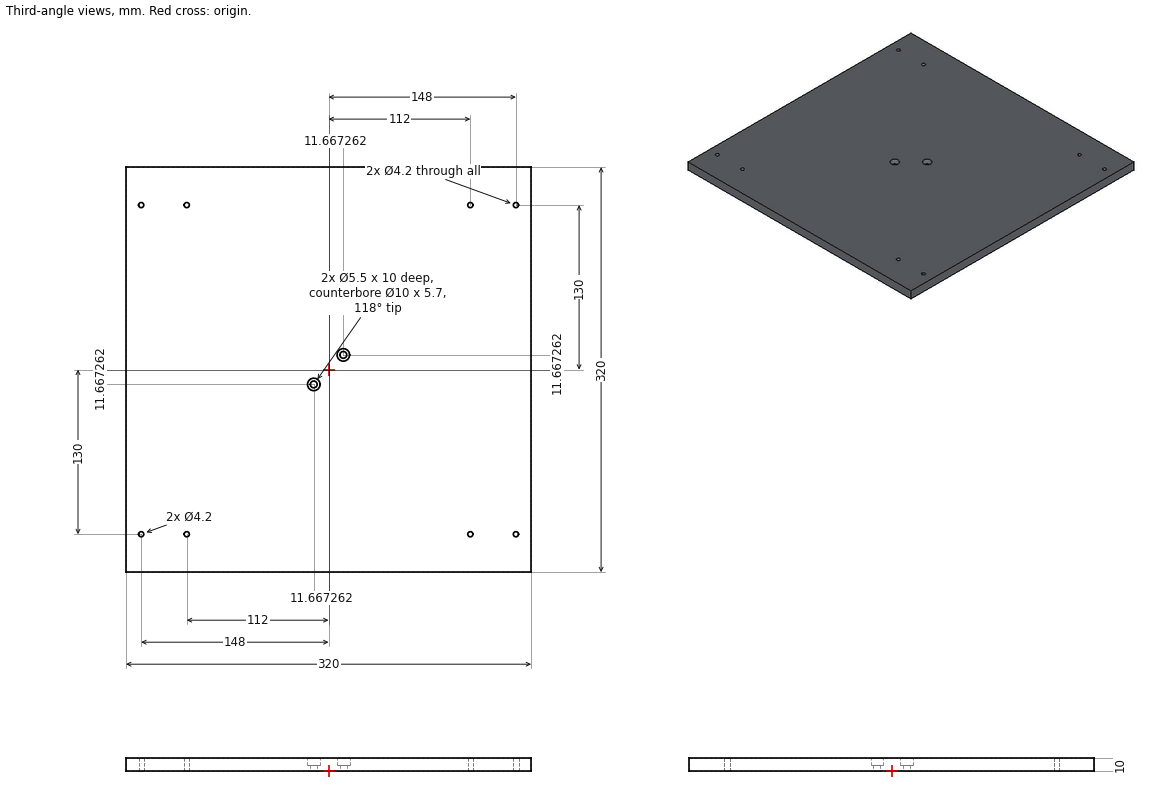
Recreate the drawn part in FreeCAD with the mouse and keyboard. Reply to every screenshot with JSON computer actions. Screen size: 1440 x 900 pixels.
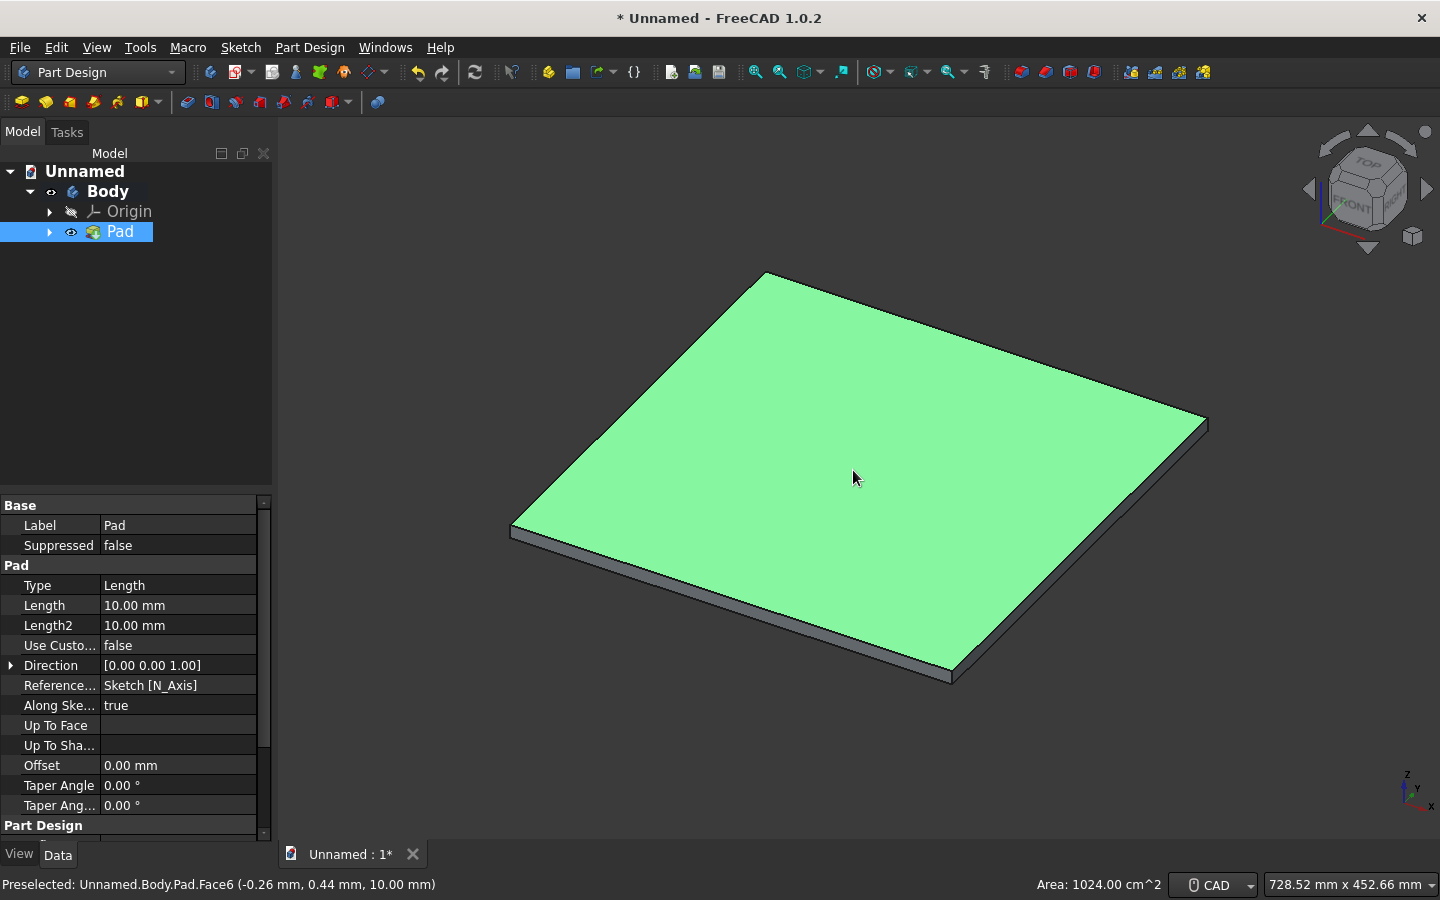
{"action": "left_click", "coordinate": [236, 72]}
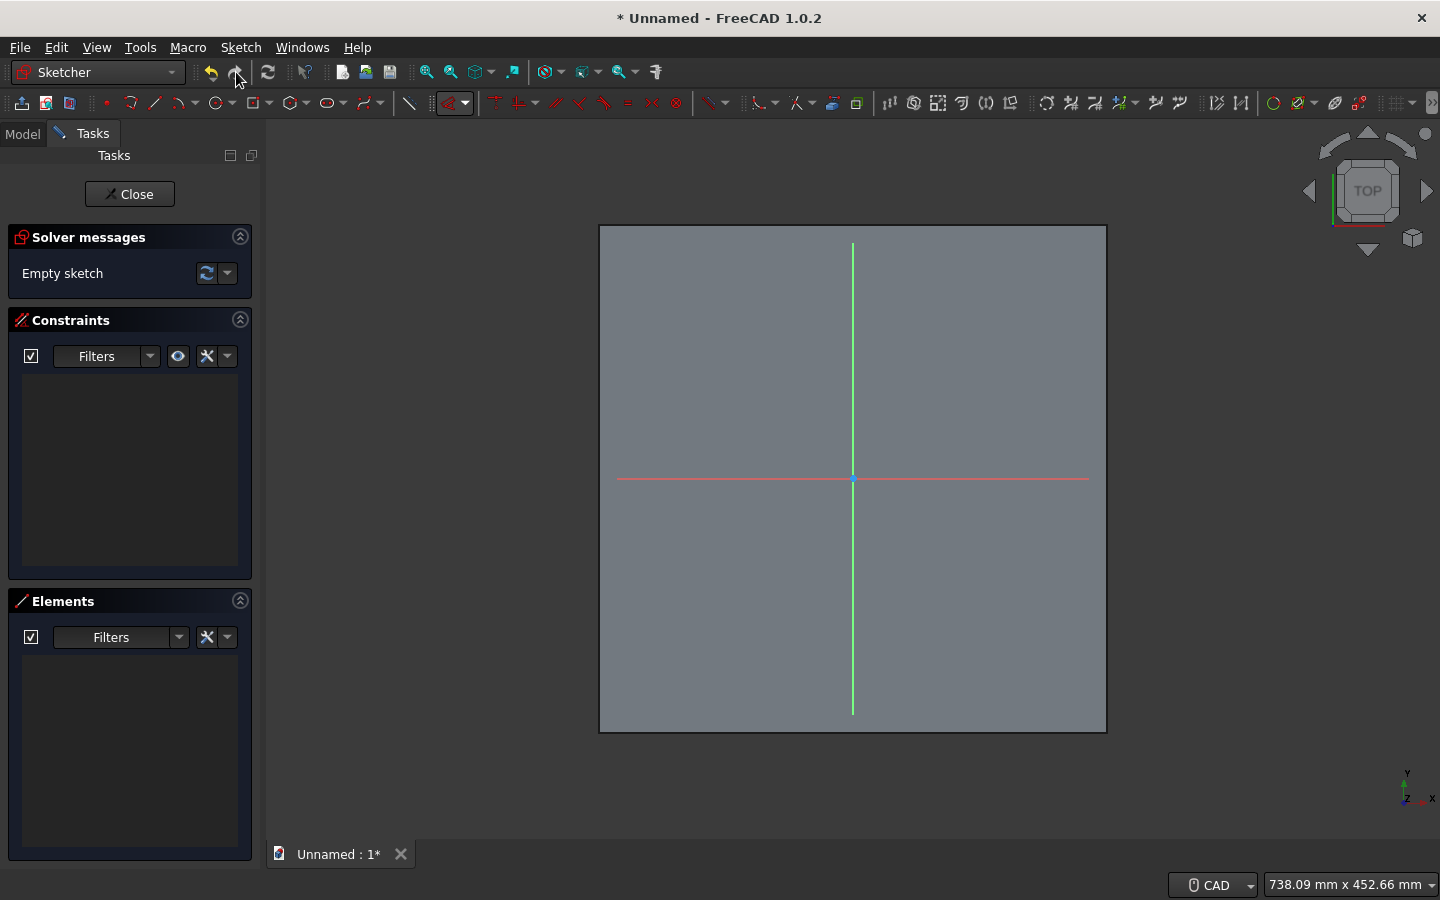
{"action": "scroll", "coordinate": [860, 479], "scroll_direction": "up", "scroll_amount": 12}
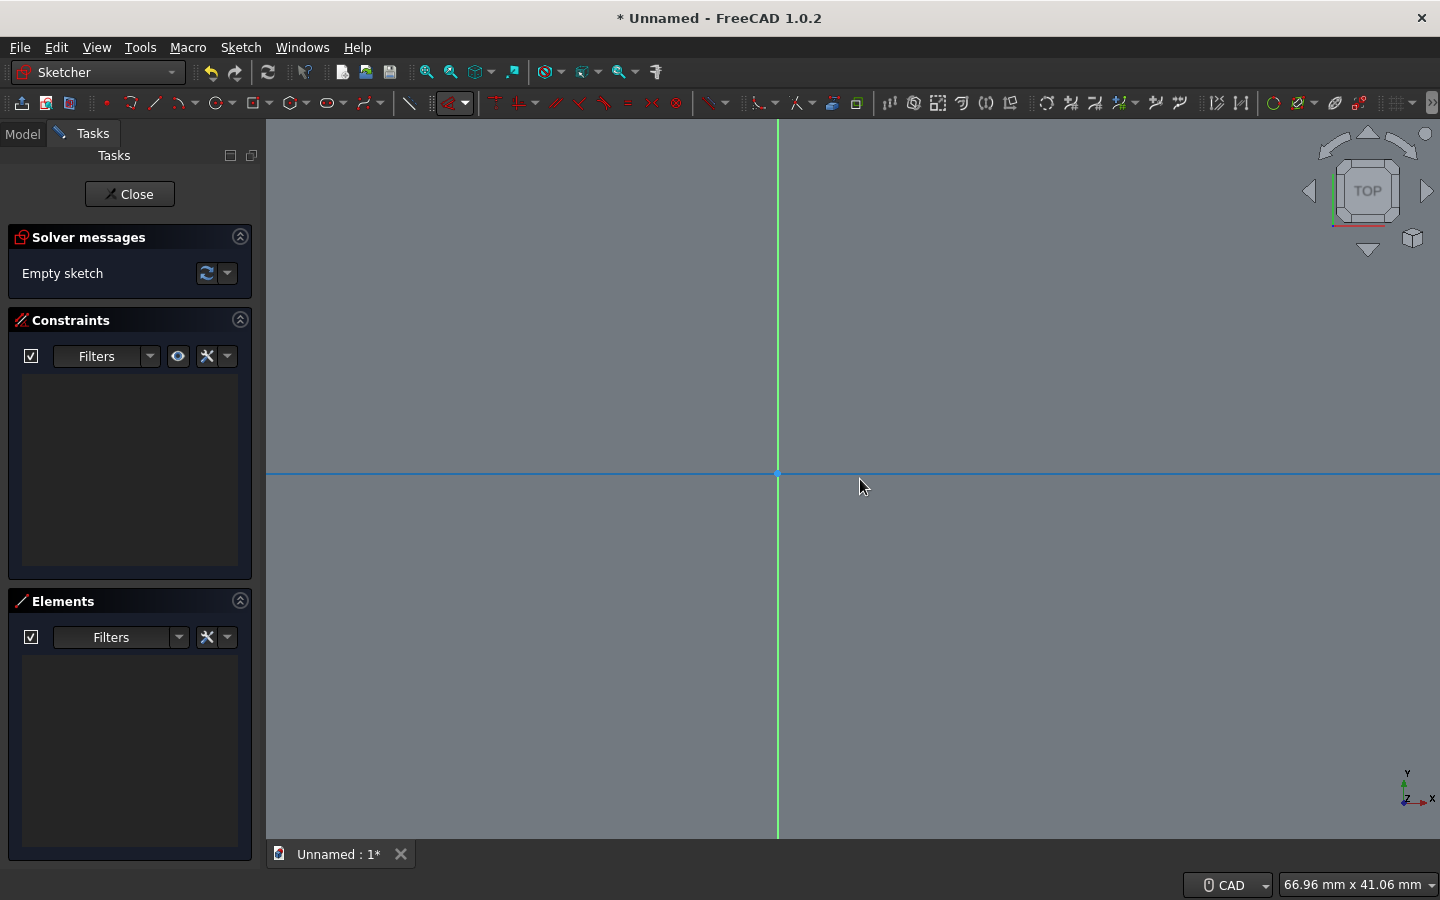
{"action": "left_click", "coordinate": [216, 104]}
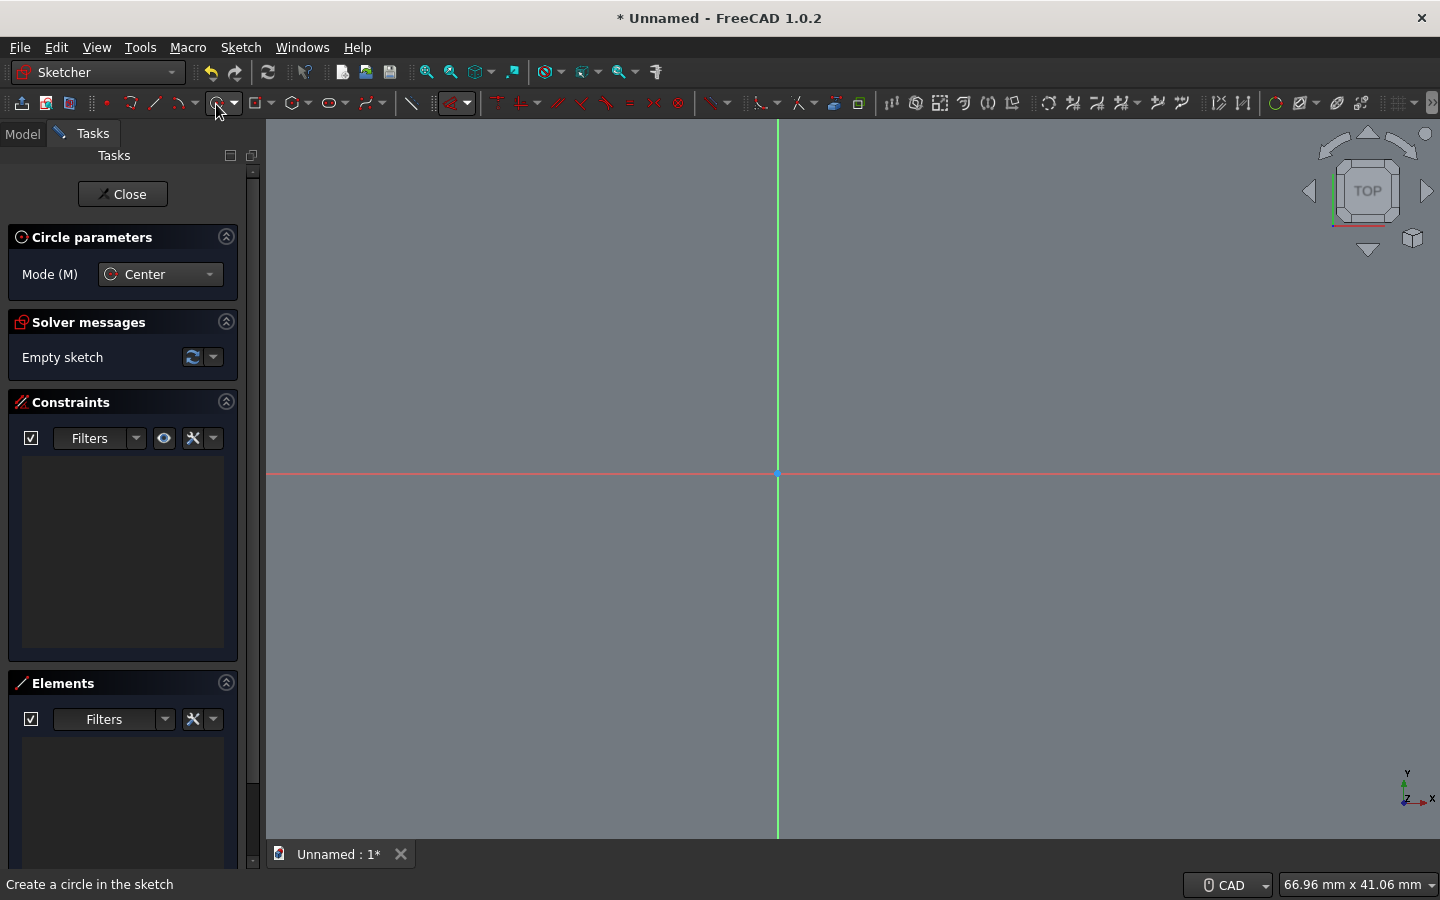
{"action": "left_click", "coordinate": [573, 679]}
{"action": "mouse_move", "coordinate": [607, 644]}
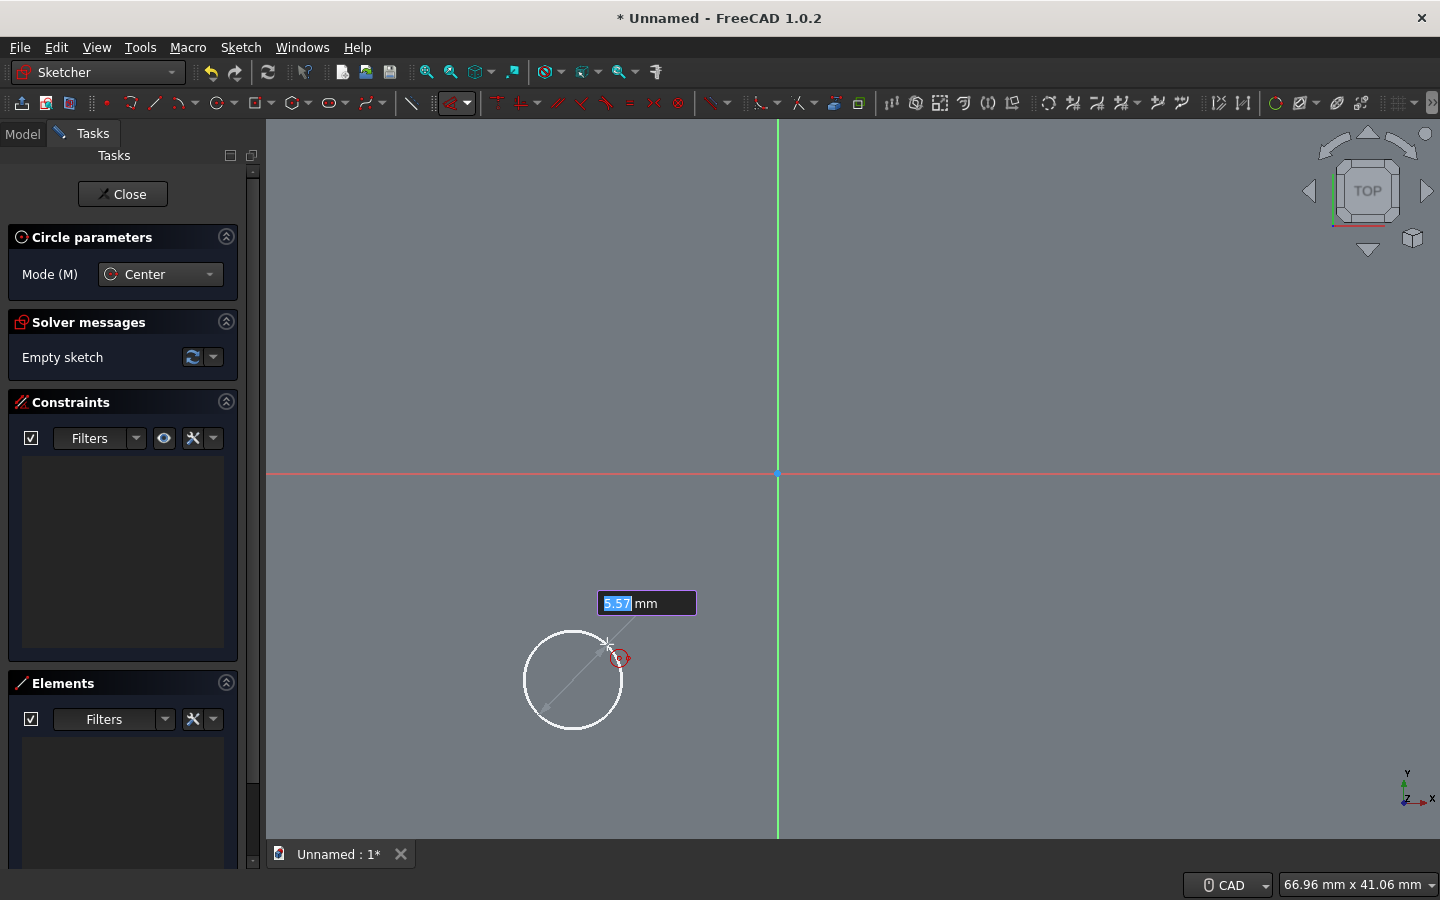
{"action": "type", "text": "5.5"}
{"action": "key", "text": "Return"}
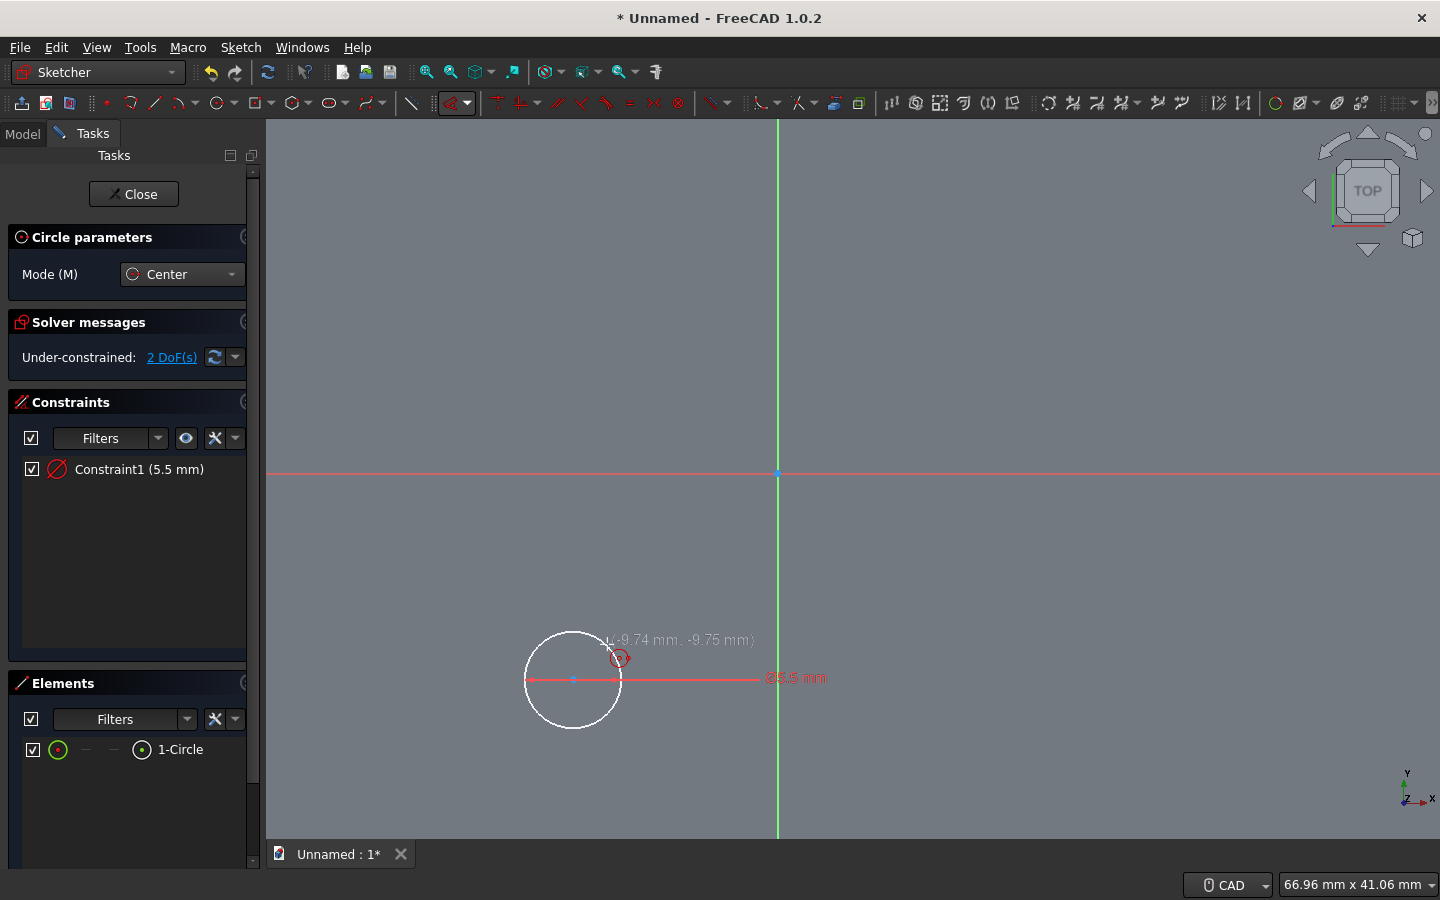
{"action": "left_click", "coordinate": [982, 269]}
{"action": "mouse_move", "coordinate": [1016, 235]}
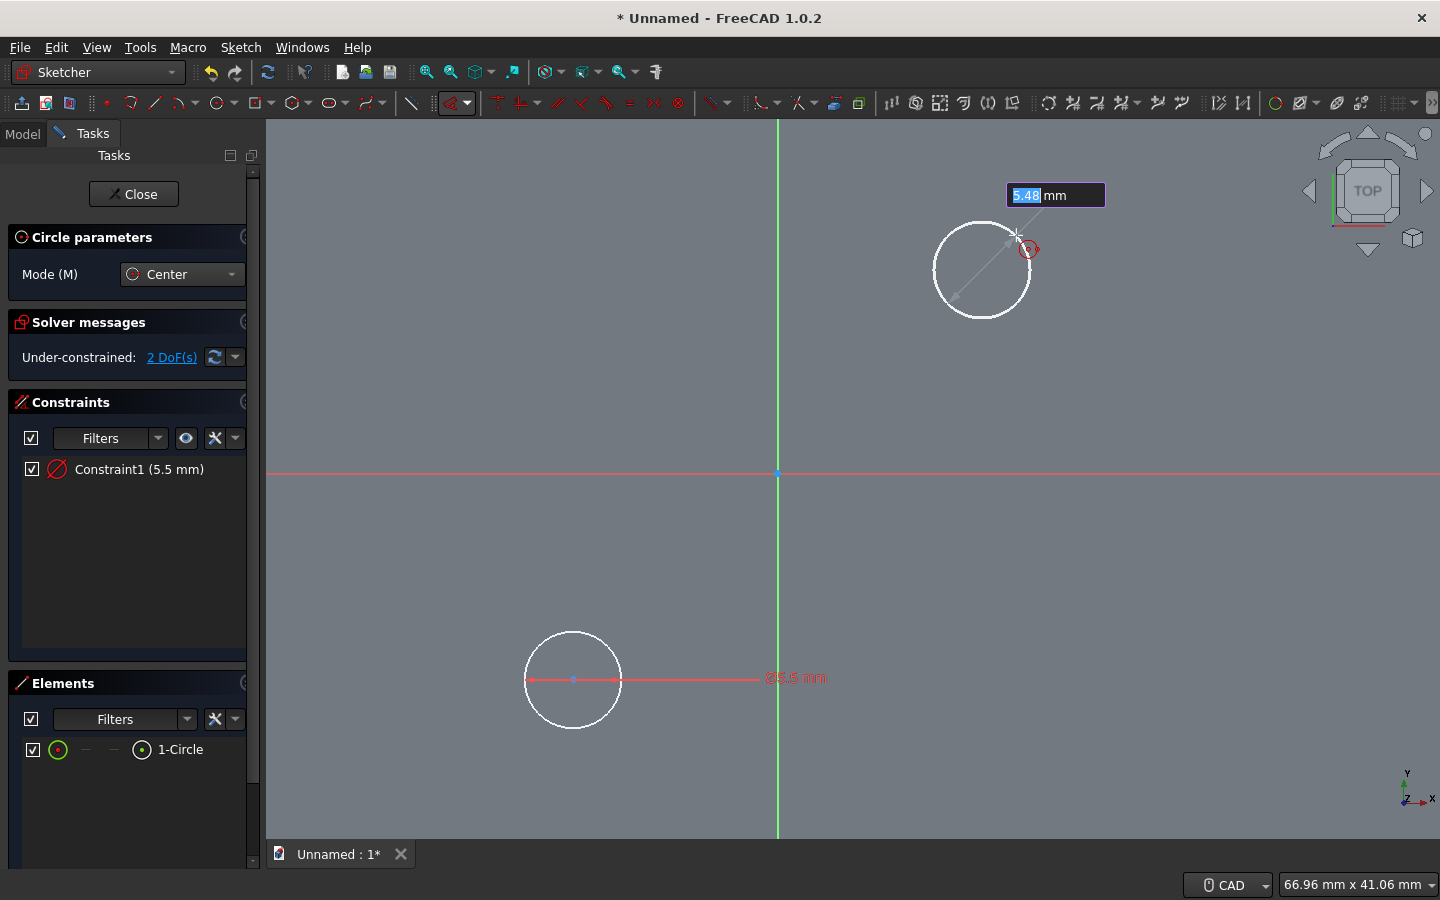
{"action": "type", "text": "5.5"}
{"action": "key", "text": "Return"}
{"action": "key", "text": "Escape"}